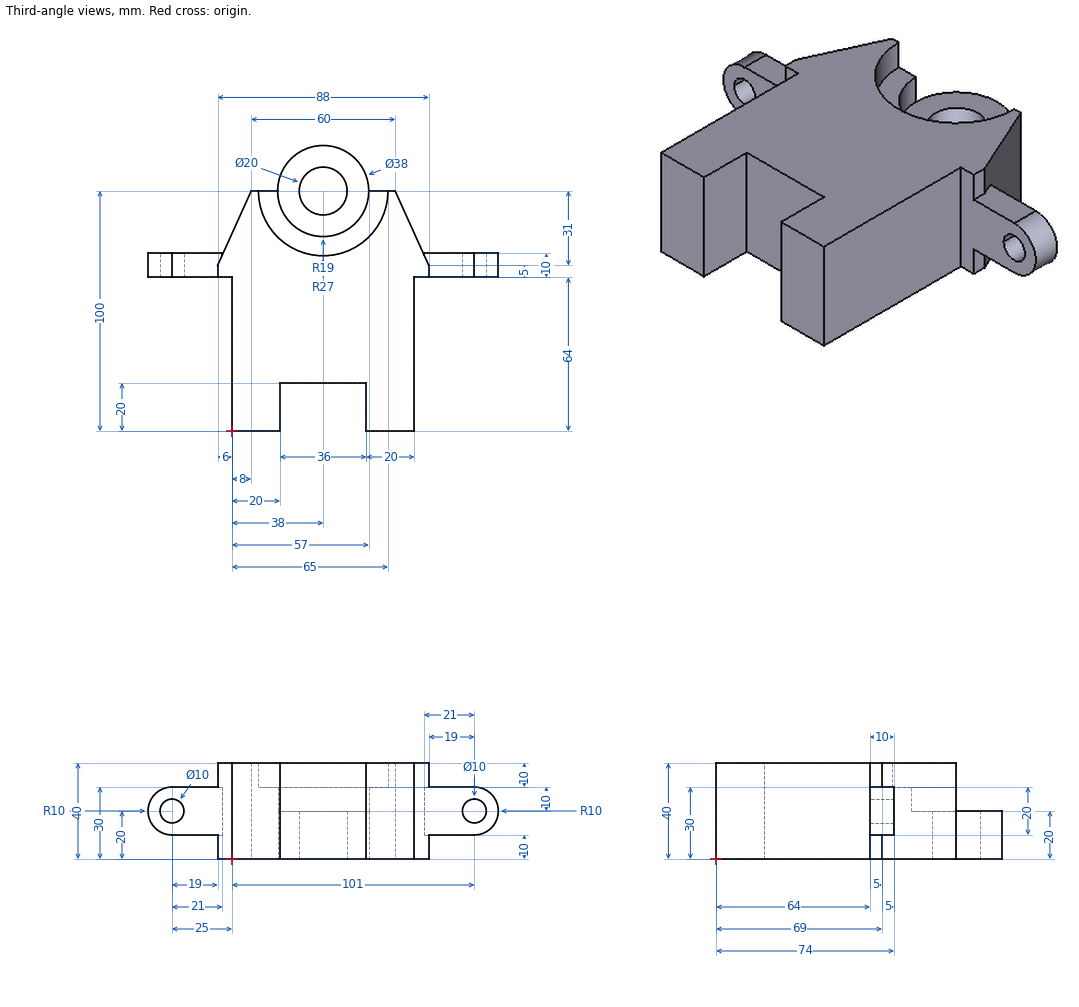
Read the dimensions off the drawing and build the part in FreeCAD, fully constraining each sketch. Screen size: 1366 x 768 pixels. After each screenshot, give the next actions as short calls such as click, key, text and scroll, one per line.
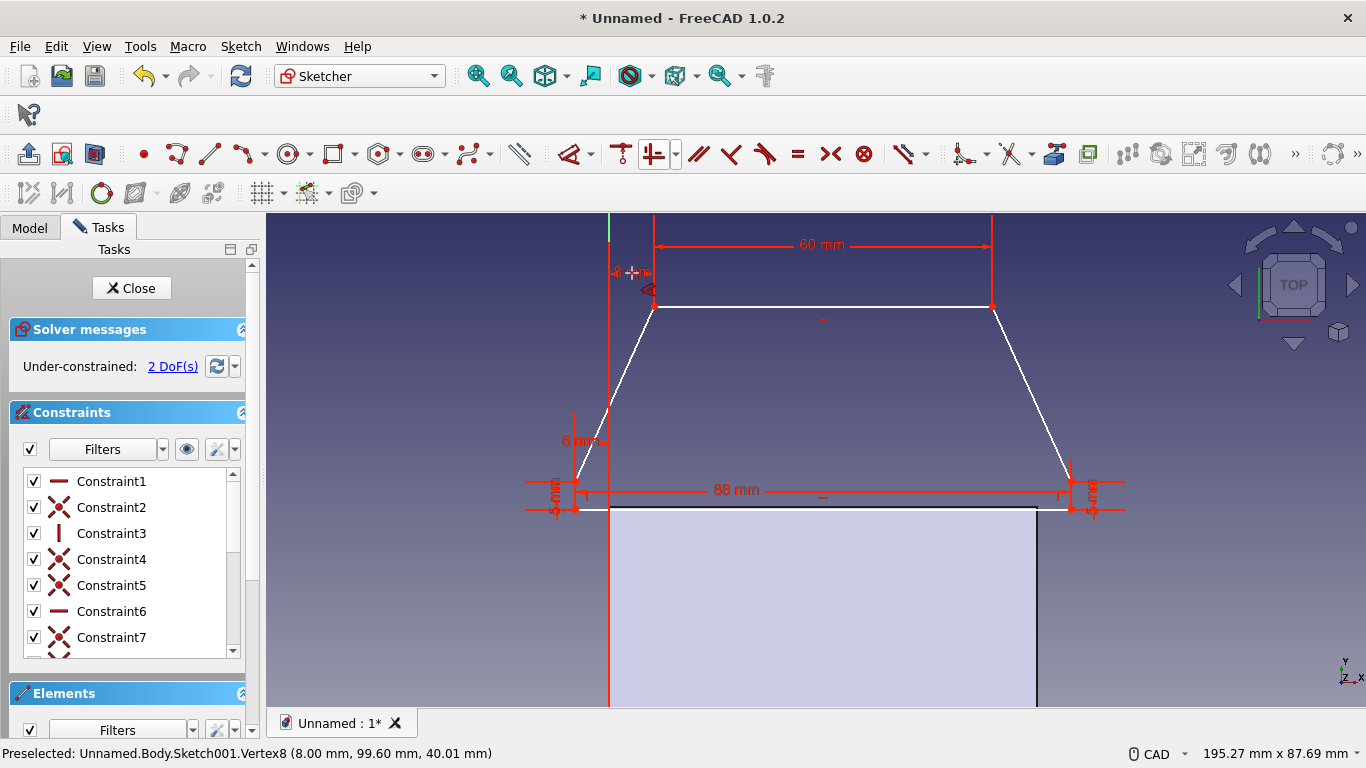
click(575, 510)
click(541, 594)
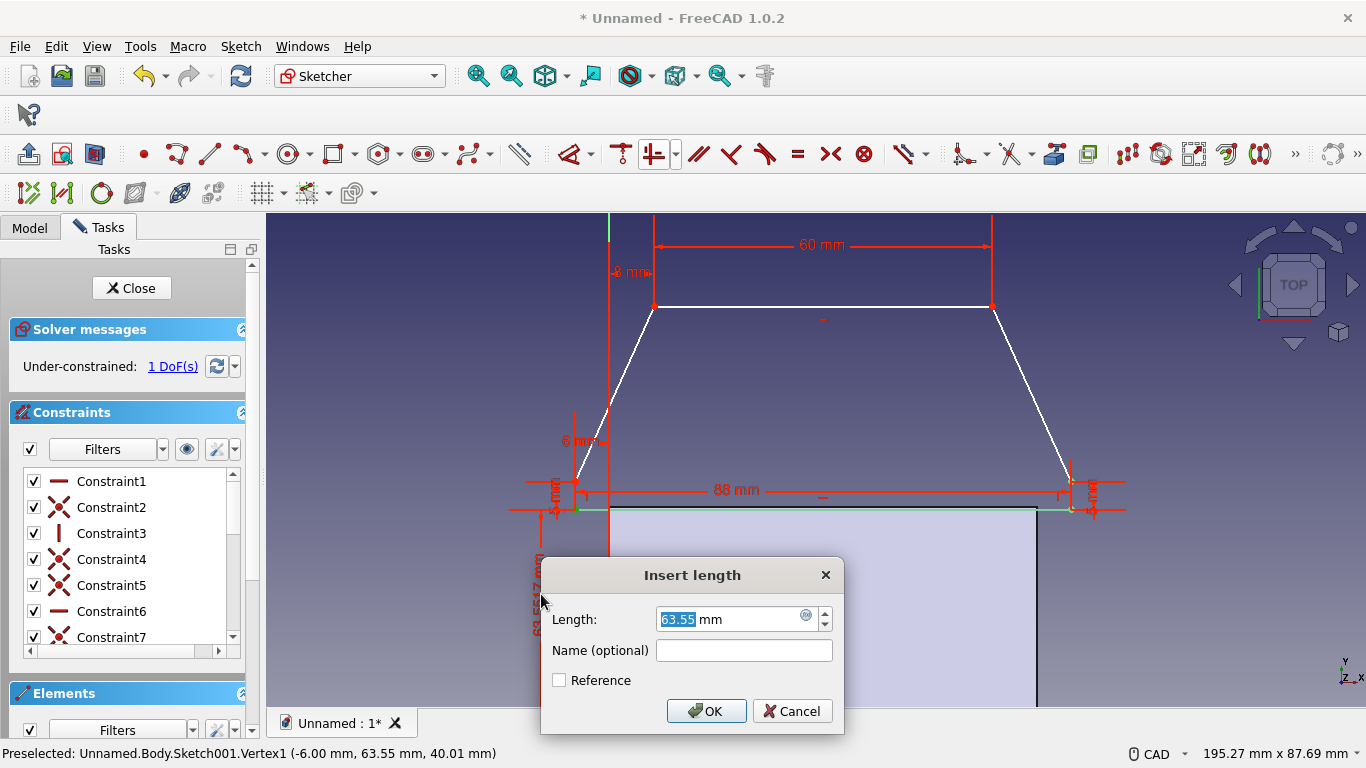
text(64)
key(Return)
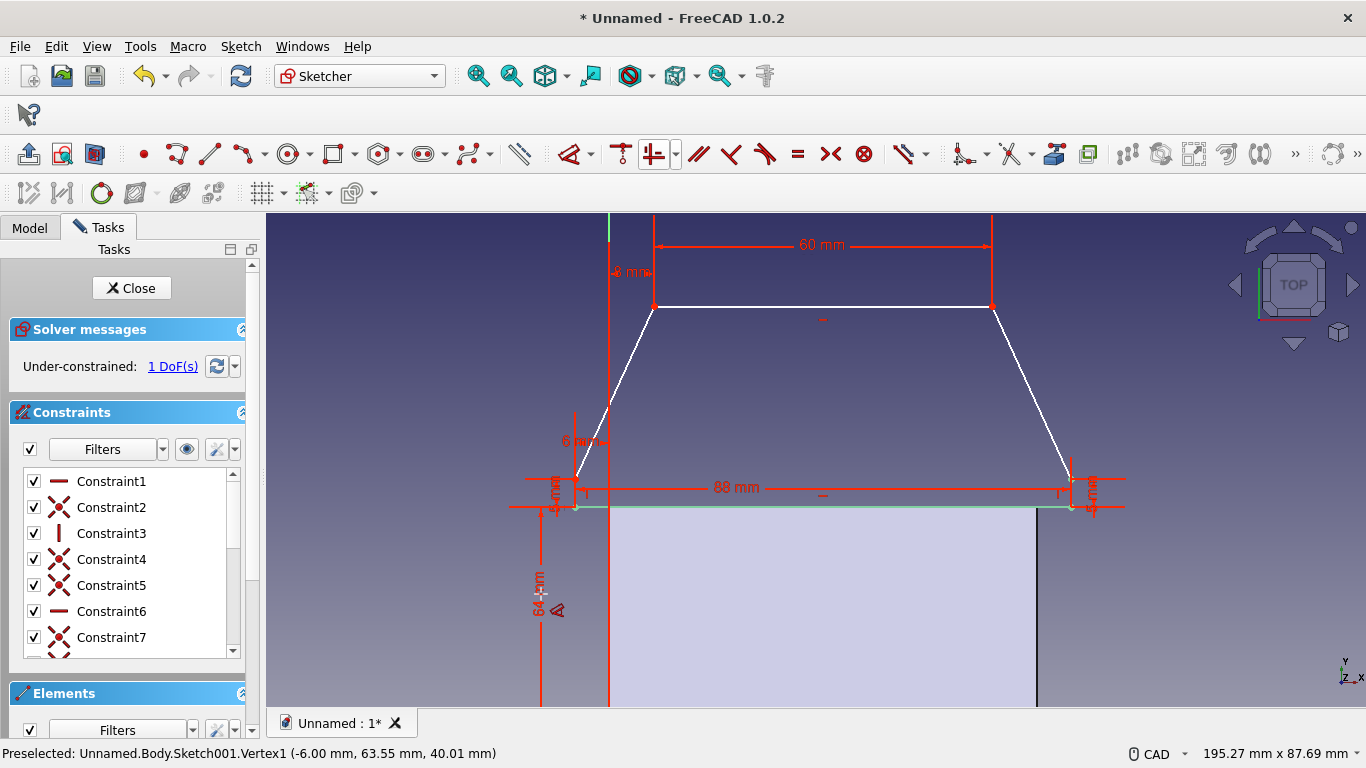
click(1047, 428)
click(1105, 393)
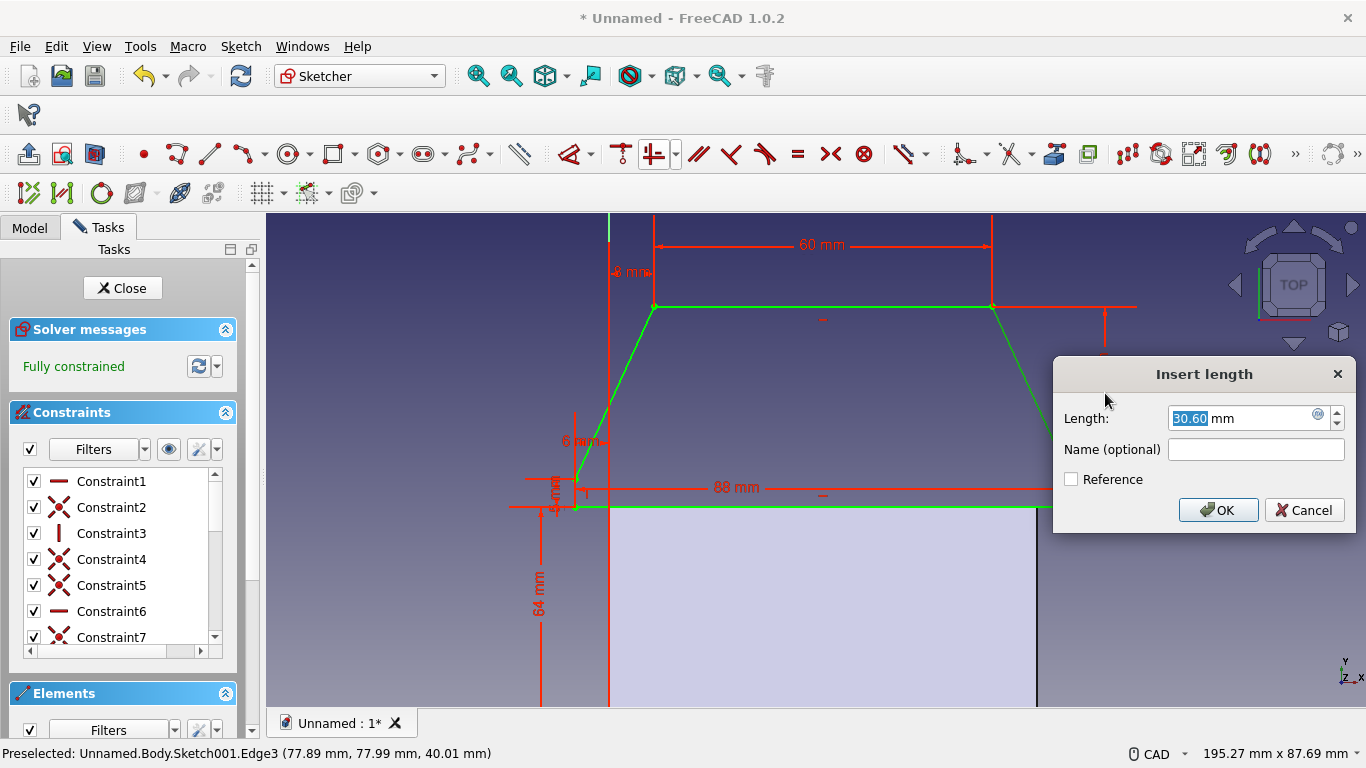
text(31)
key(Return)
key(Escape)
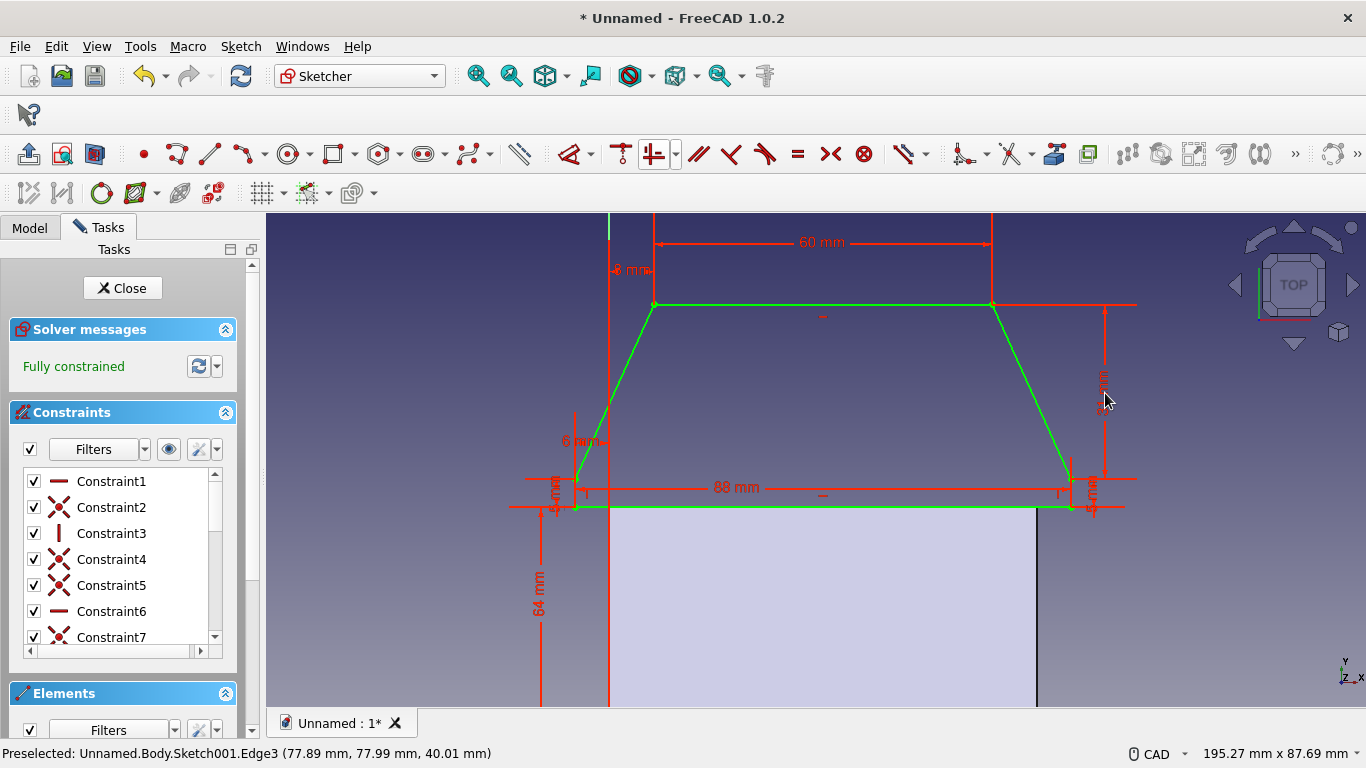
click(123, 288)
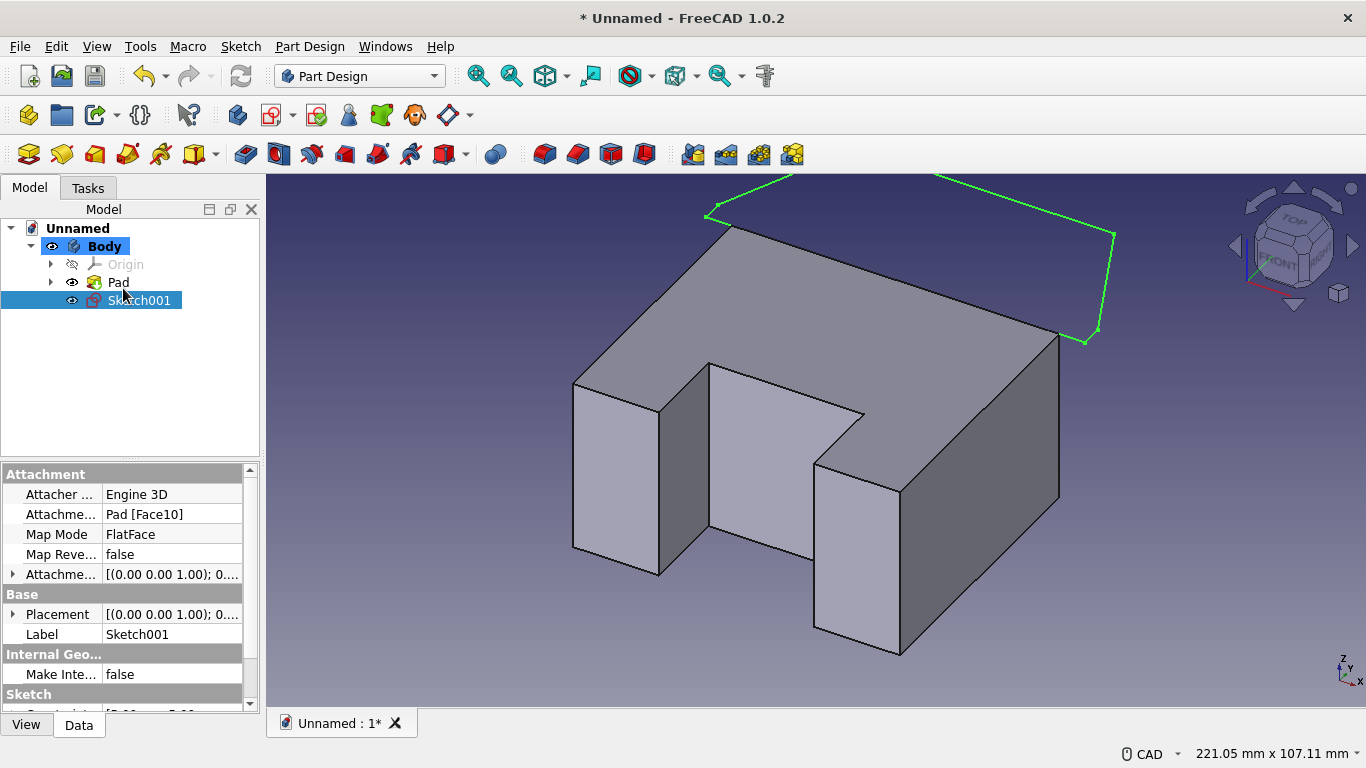
click(29, 154)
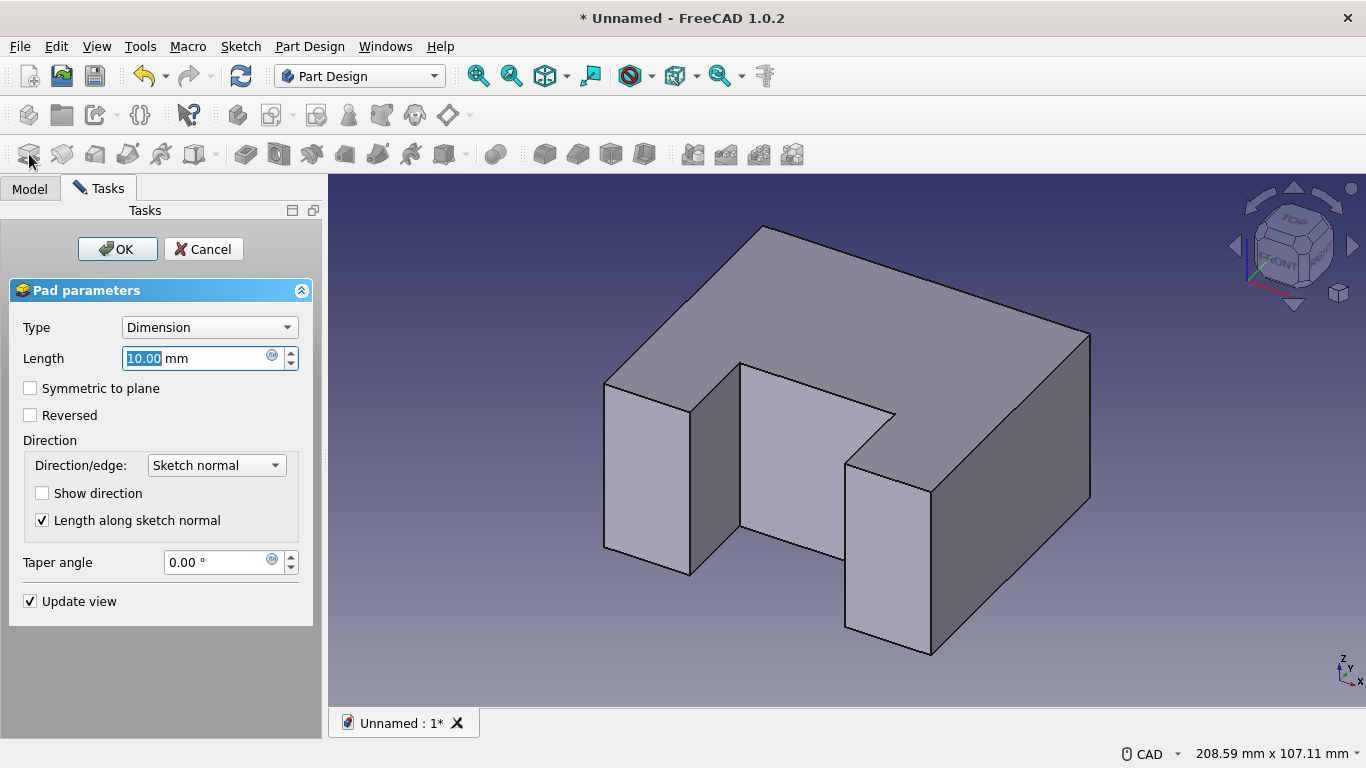
text(40)
key(Tab)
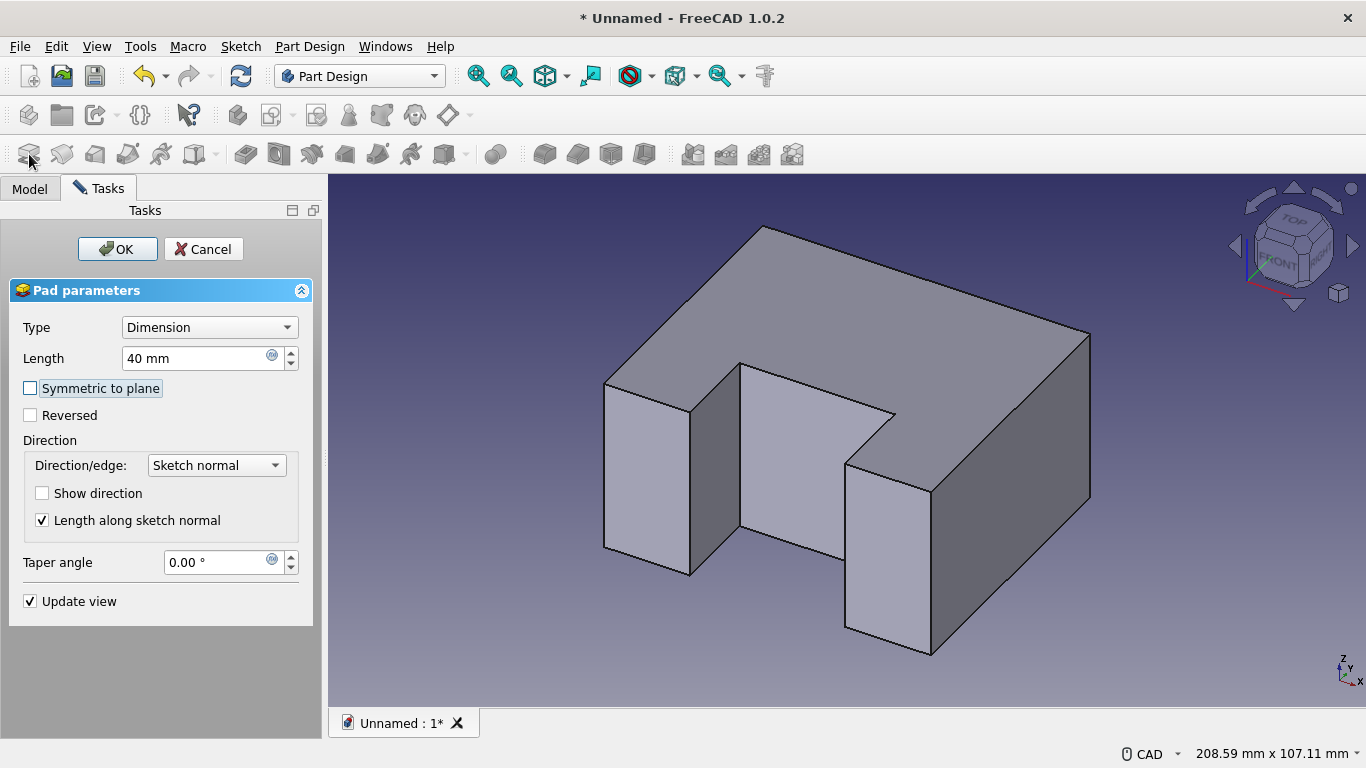
click(31, 415)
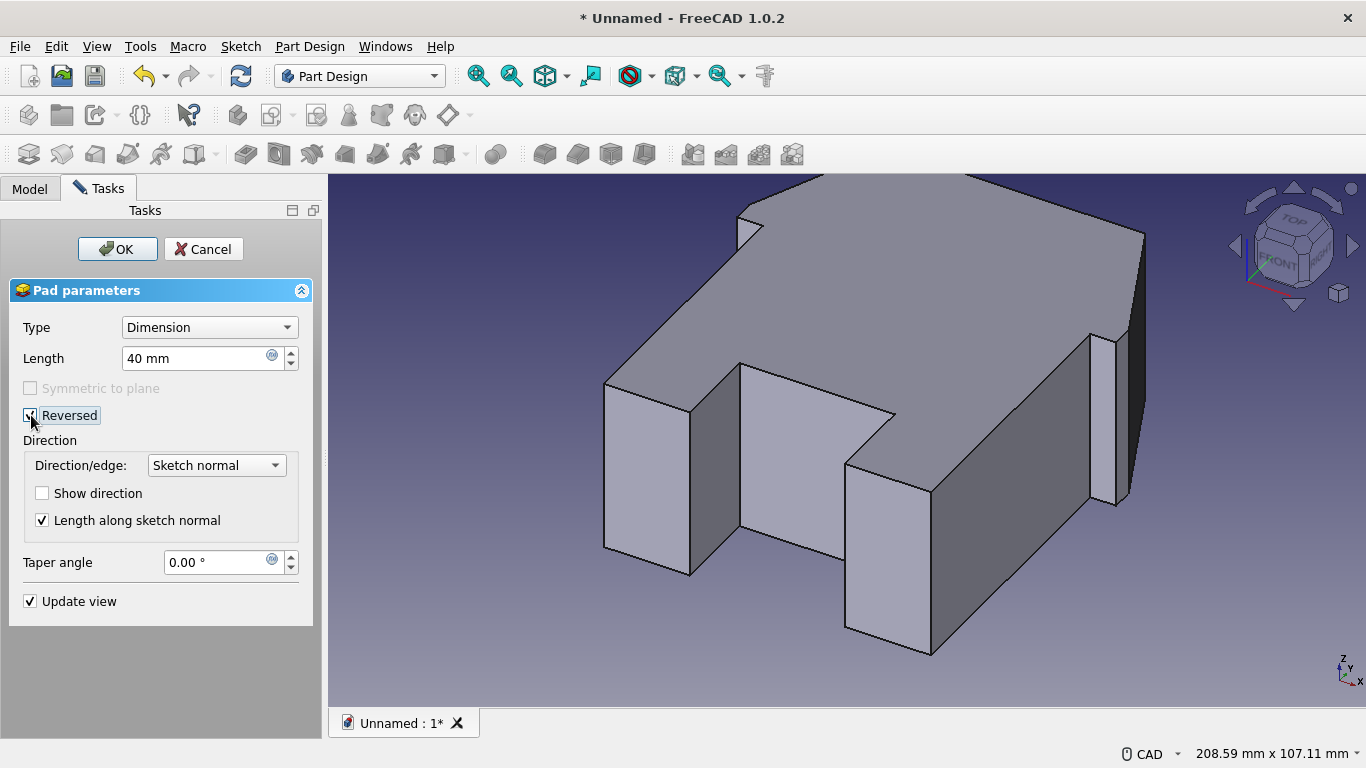
click(118, 249)